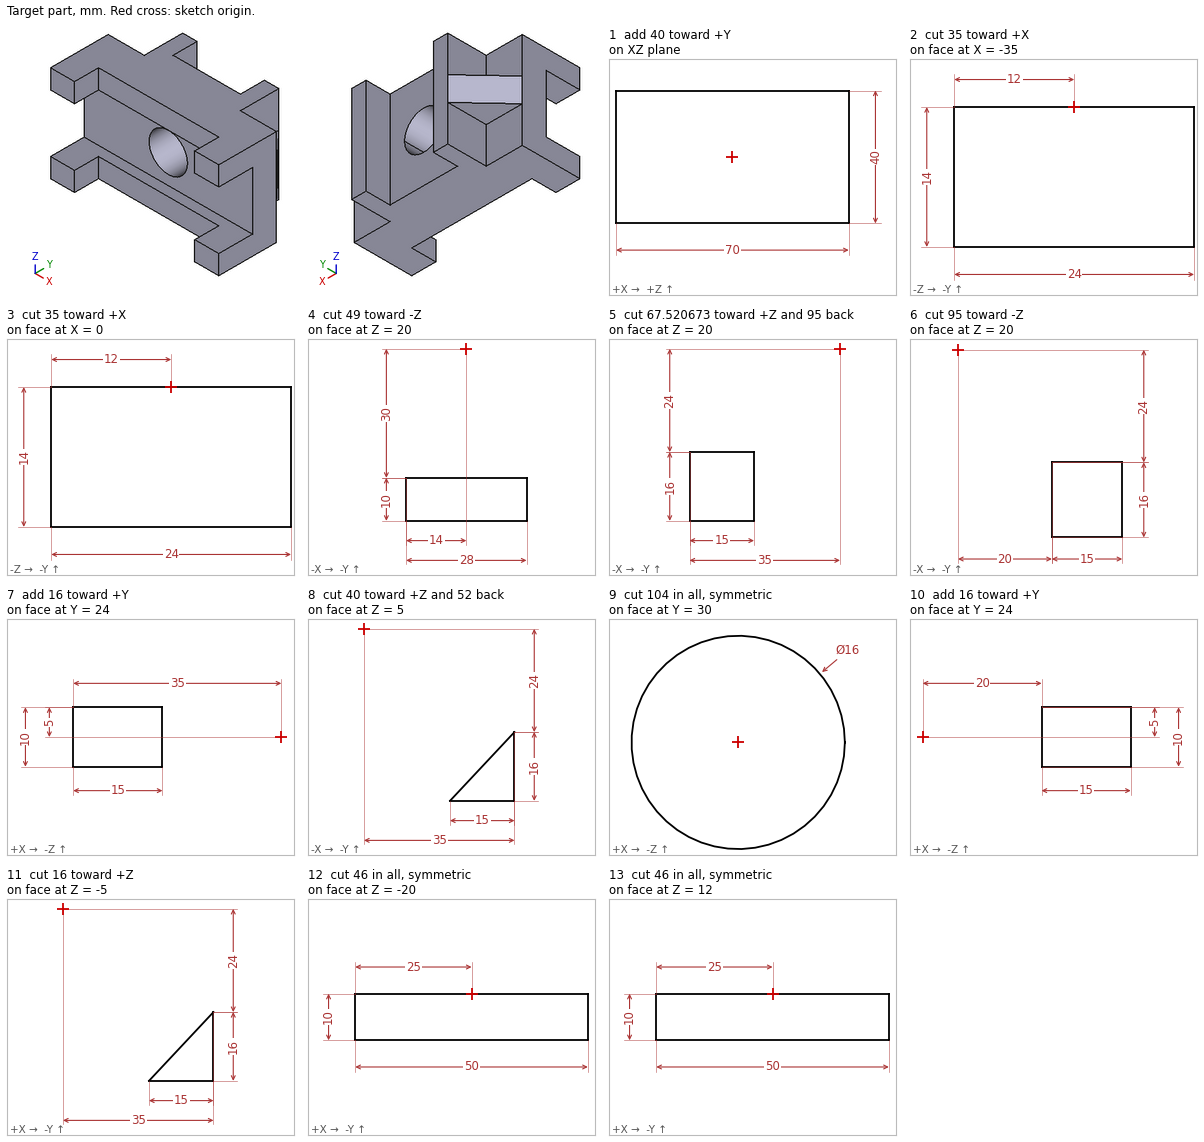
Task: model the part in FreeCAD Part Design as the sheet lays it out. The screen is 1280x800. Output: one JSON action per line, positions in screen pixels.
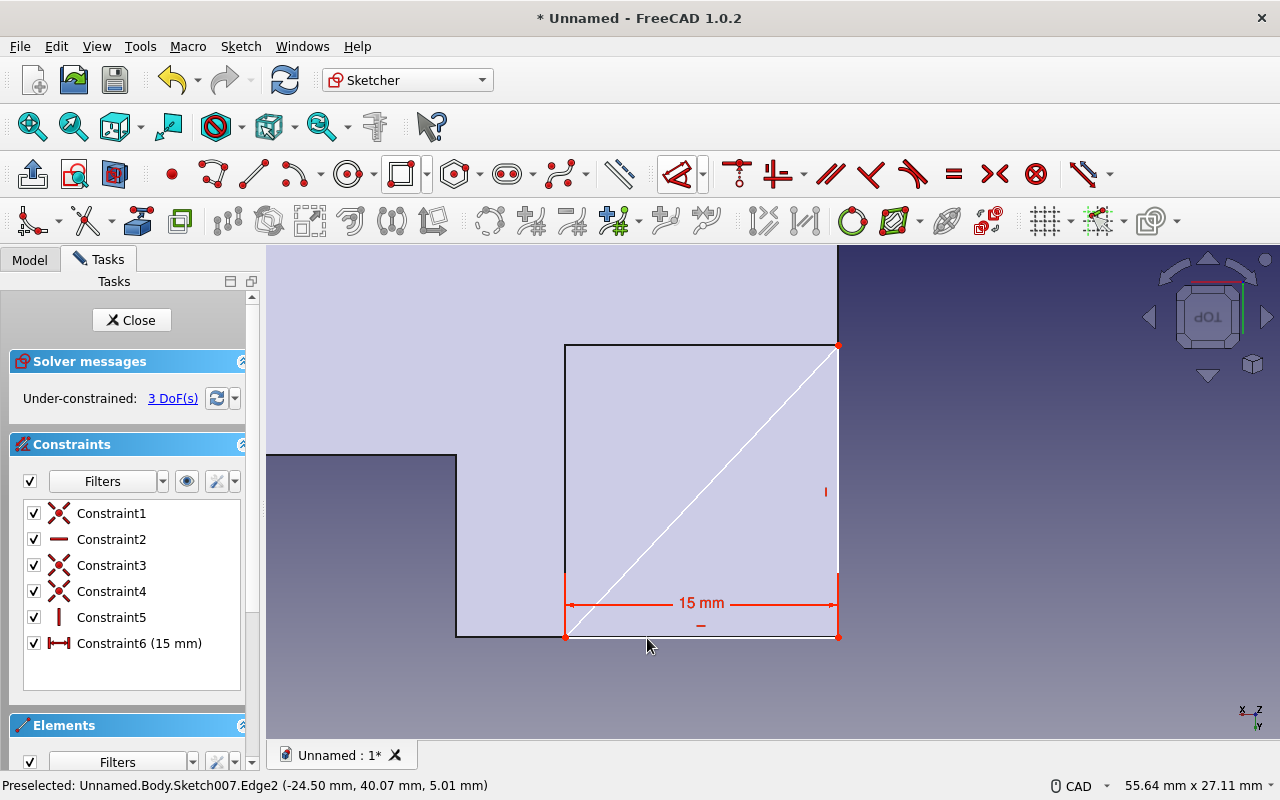
{"action": "left_click", "coordinate": [838, 550]}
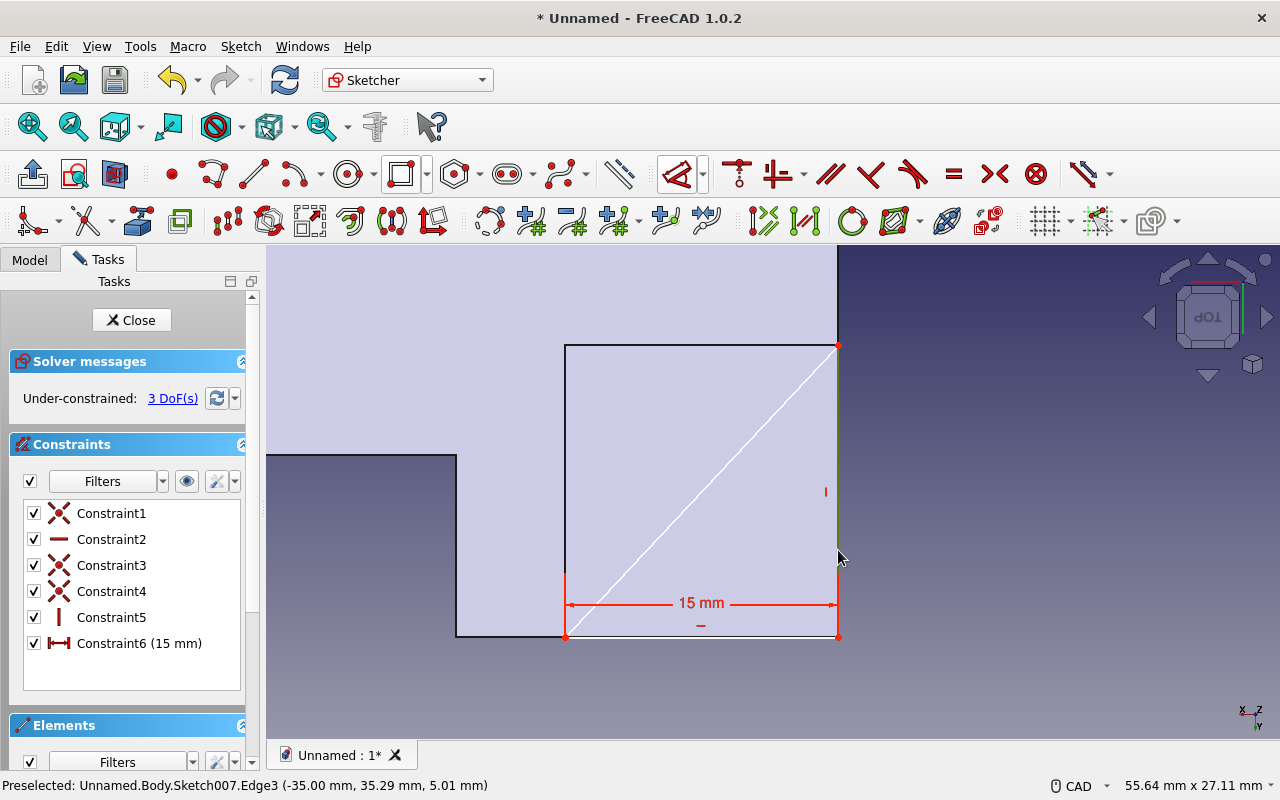
{"action": "key", "text": "i"}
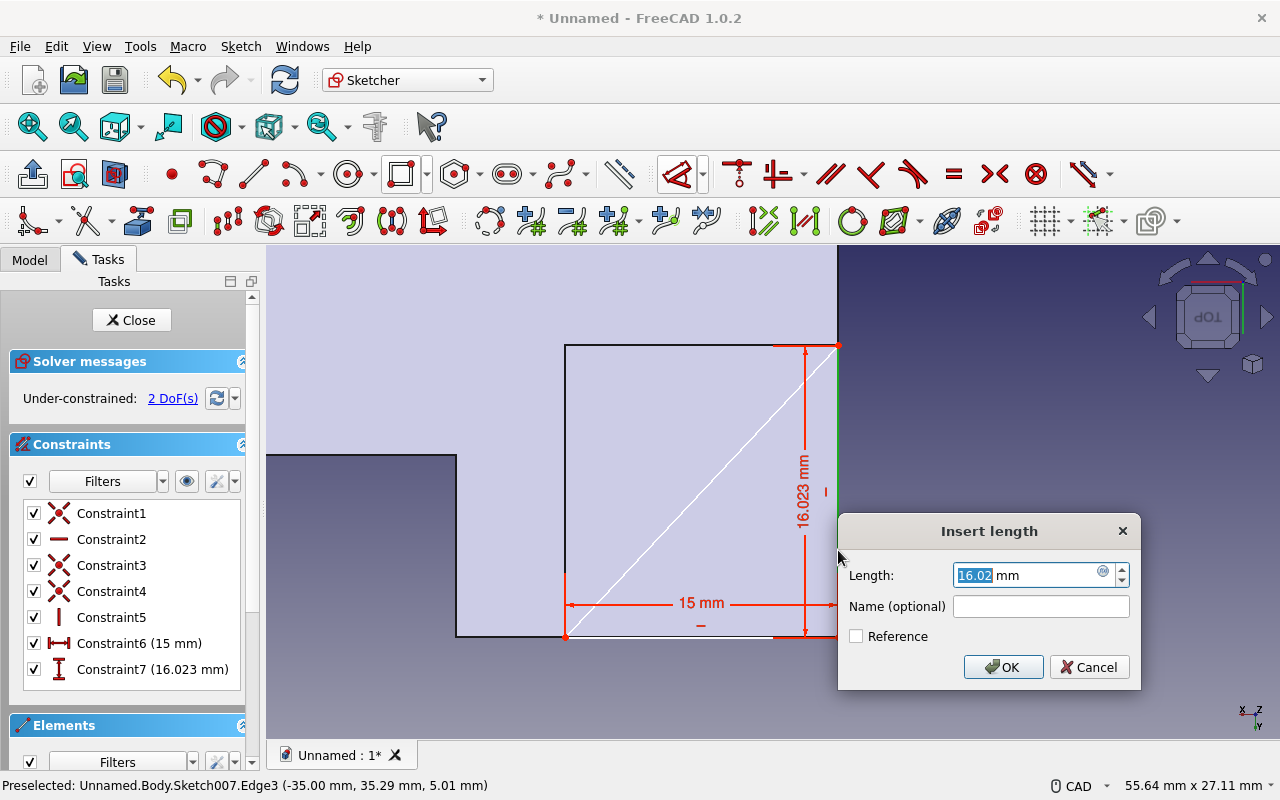
{"action": "type", "text": "16"}
{"action": "key", "text": "Return"}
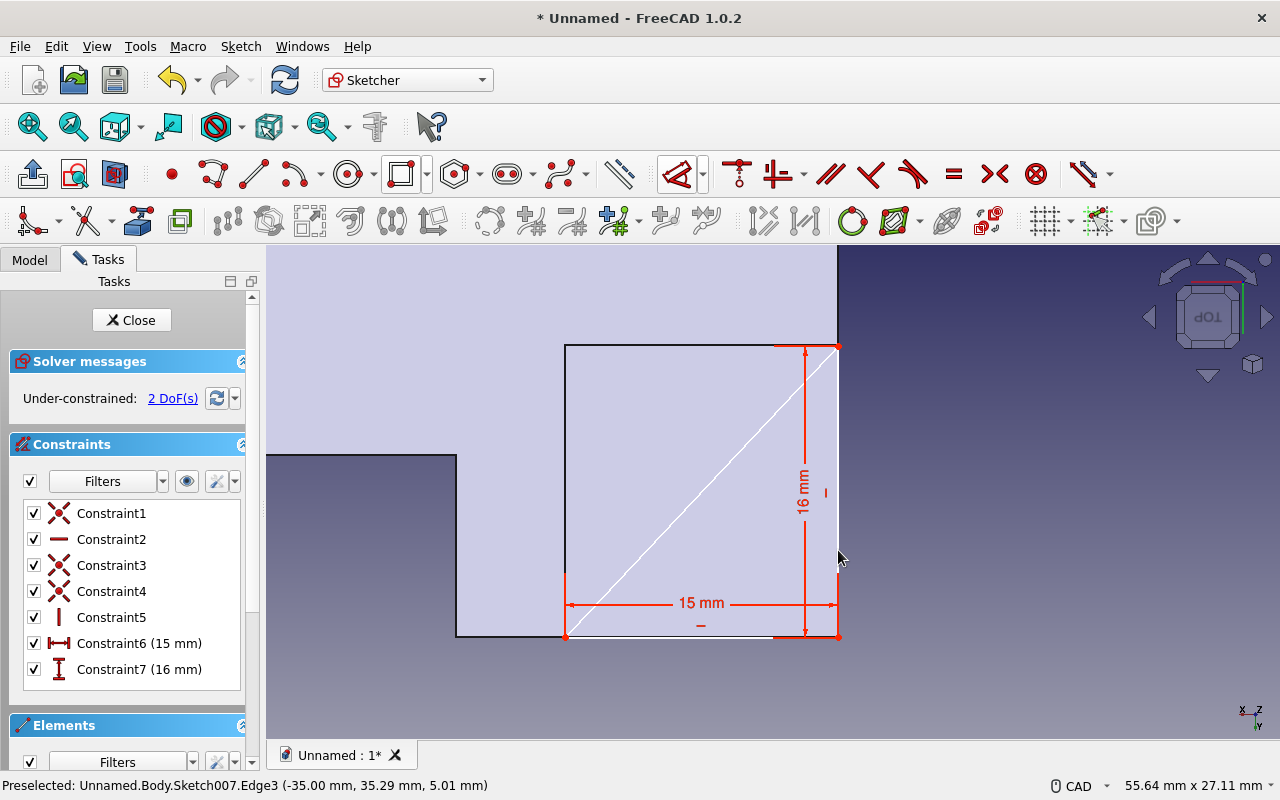
{"action": "left_click", "coordinate": [838, 346]}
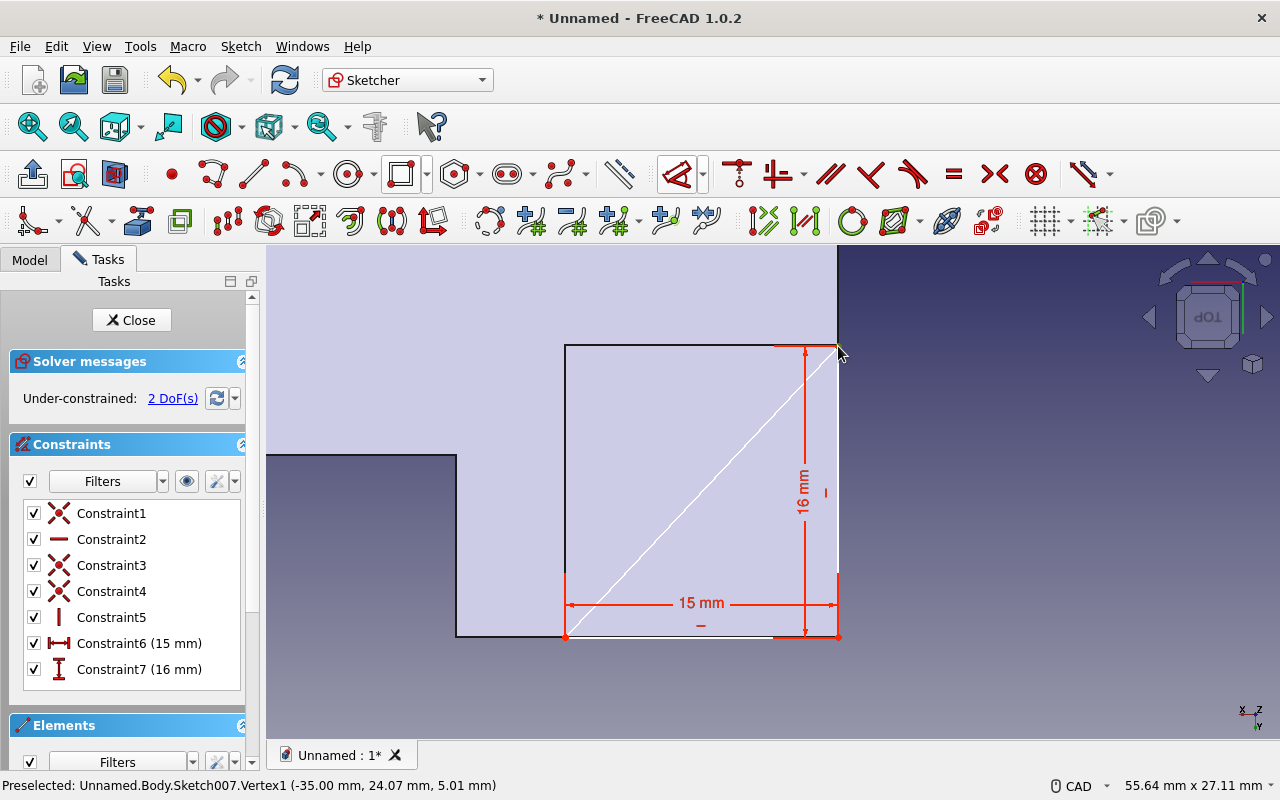
{"action": "key", "text": "l"}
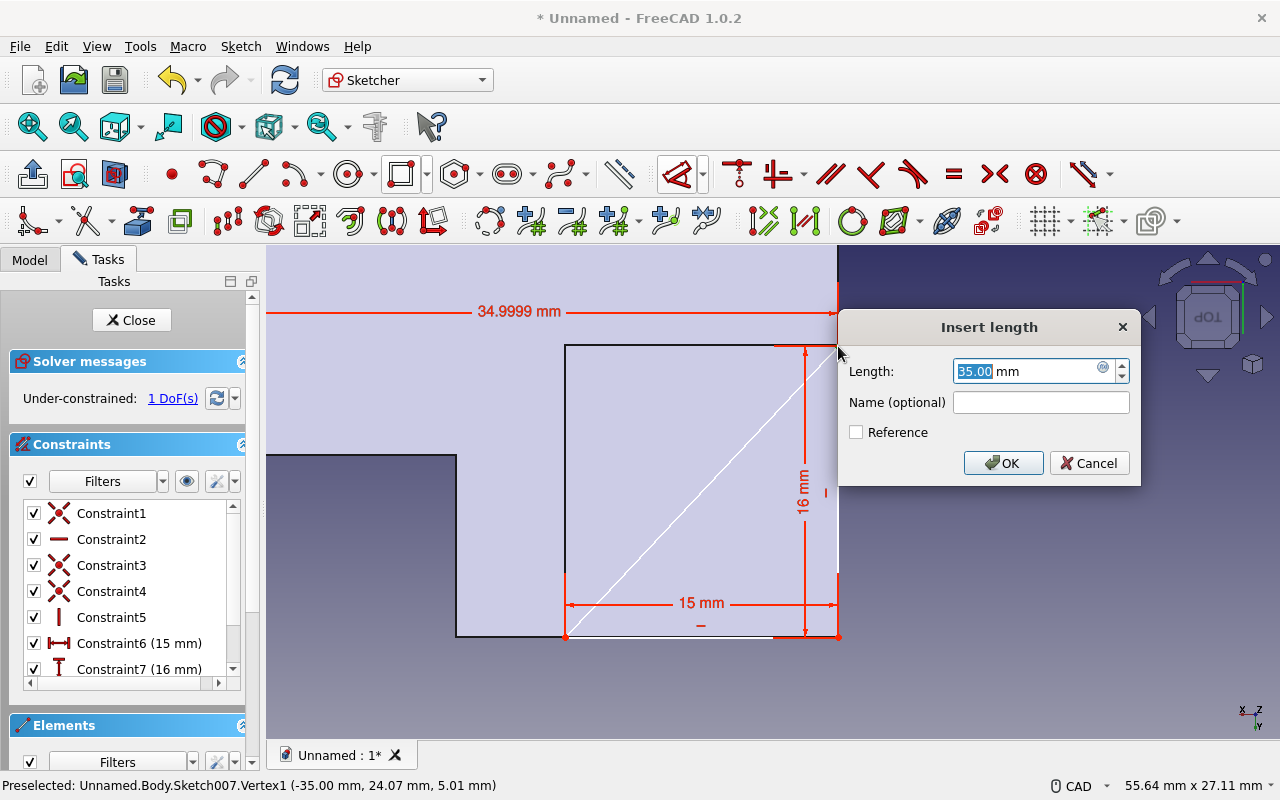
{"action": "type", "text": "35"}
{"action": "key", "text": "Return"}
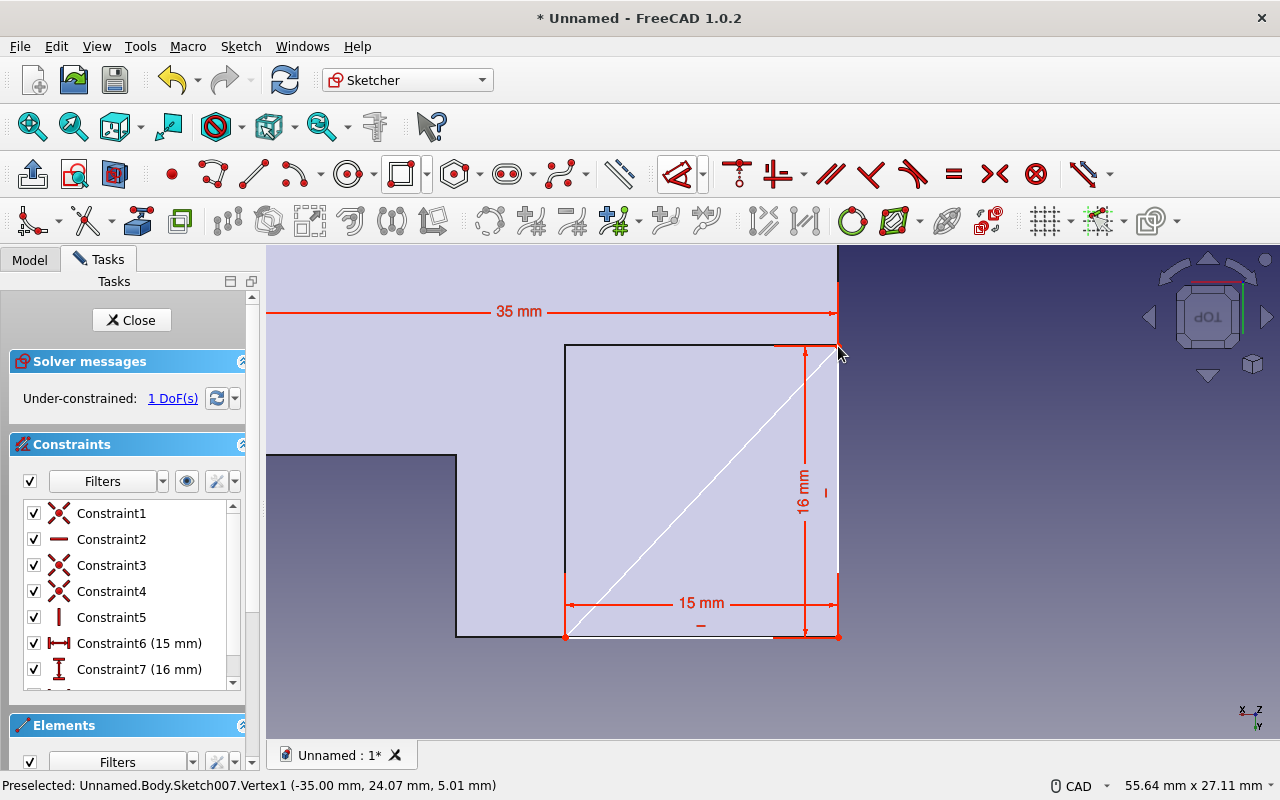
{"action": "left_click", "coordinate": [838, 346]}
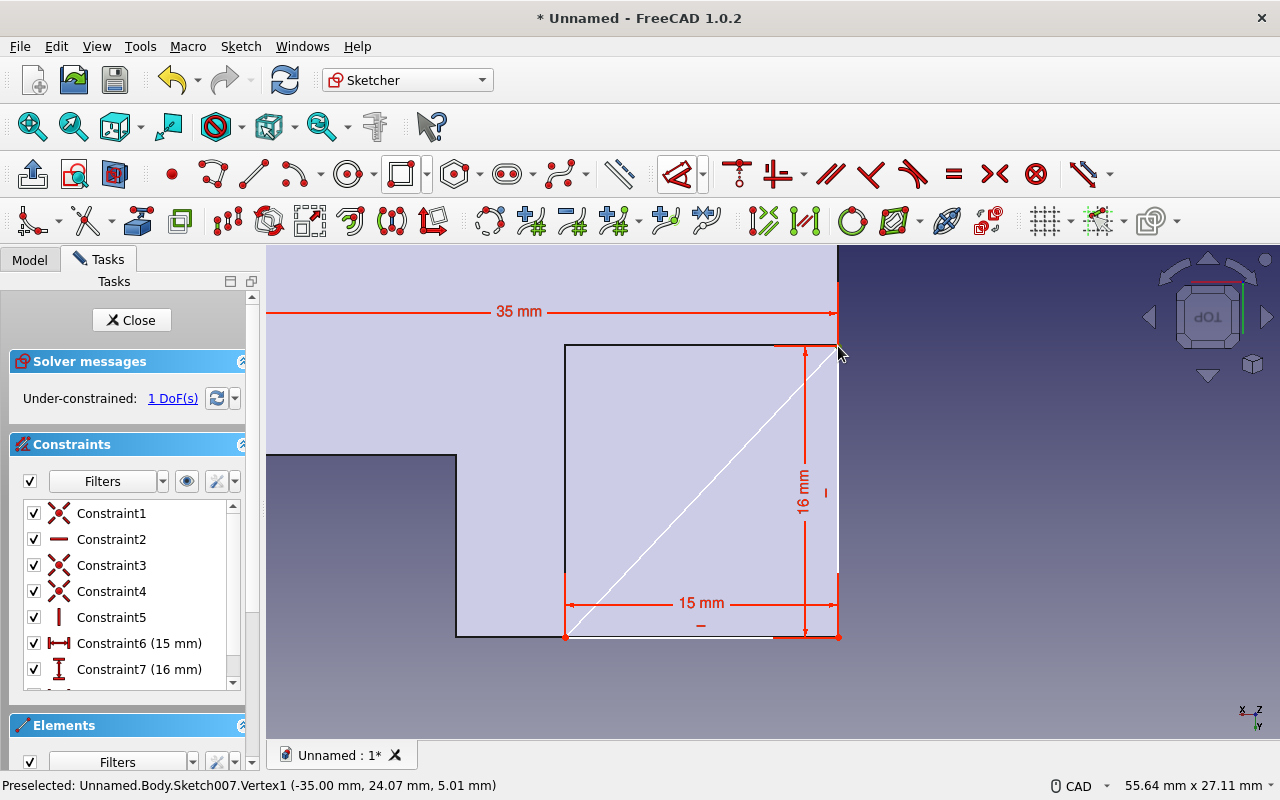
{"action": "left_click", "coordinate": [702, 174]}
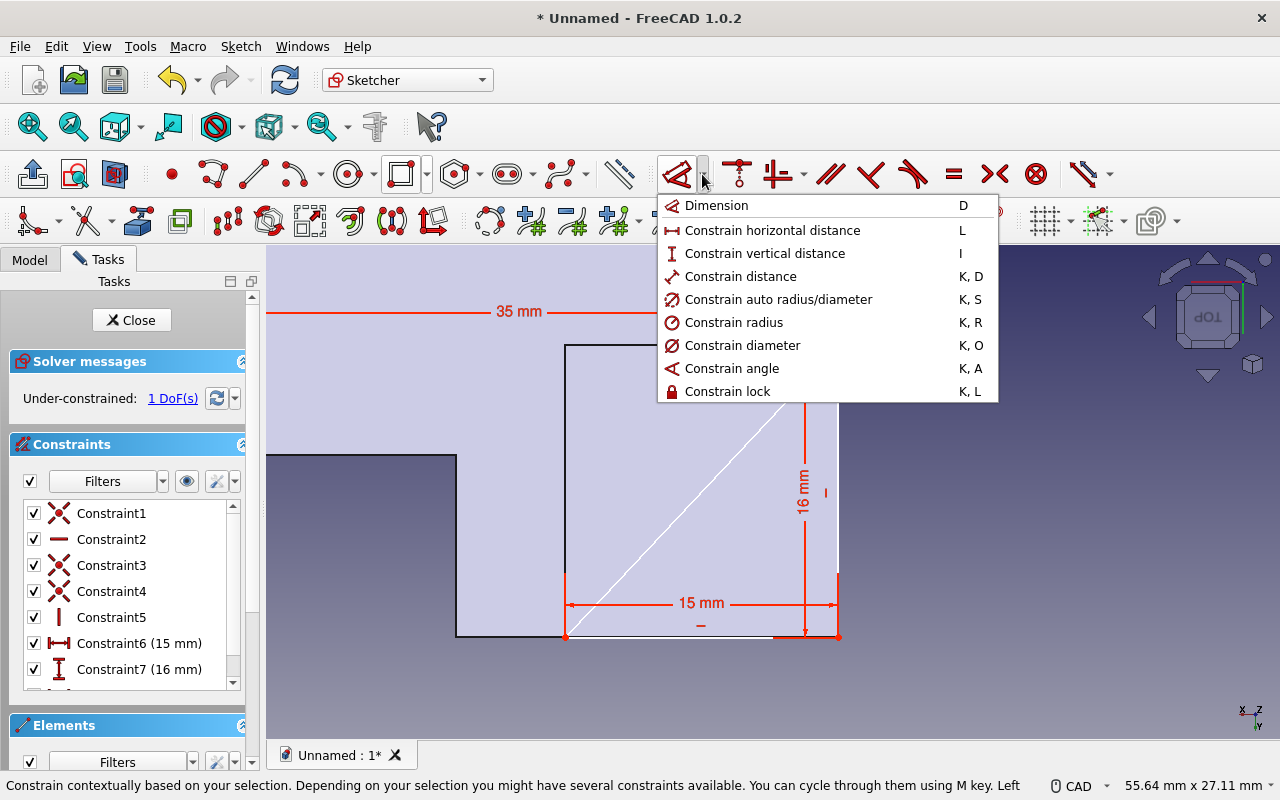
{"action": "left_click", "coordinate": [828, 254]}